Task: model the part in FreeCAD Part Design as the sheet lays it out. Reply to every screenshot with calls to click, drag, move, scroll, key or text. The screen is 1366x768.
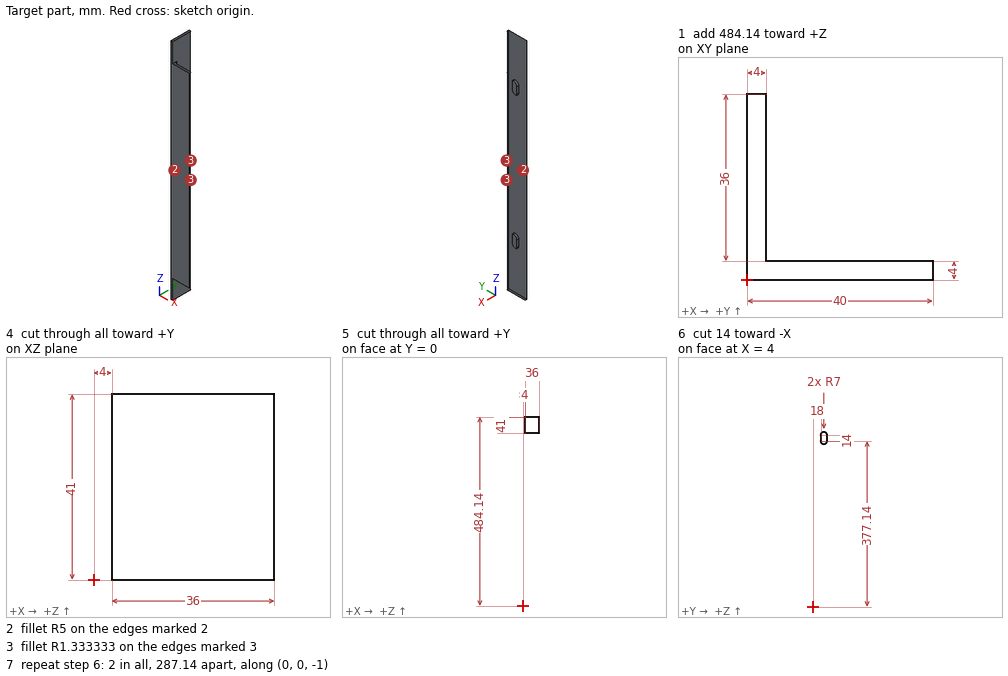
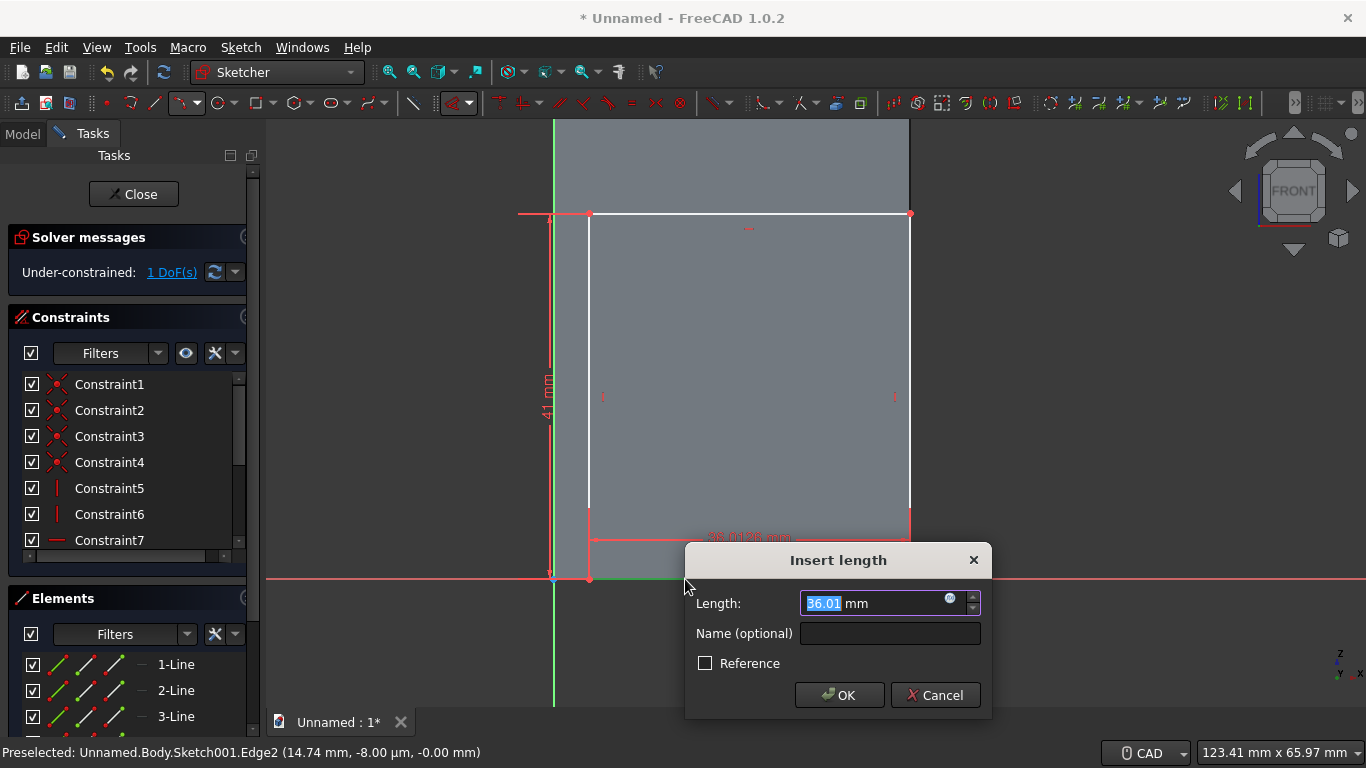
text(36)
key(Return)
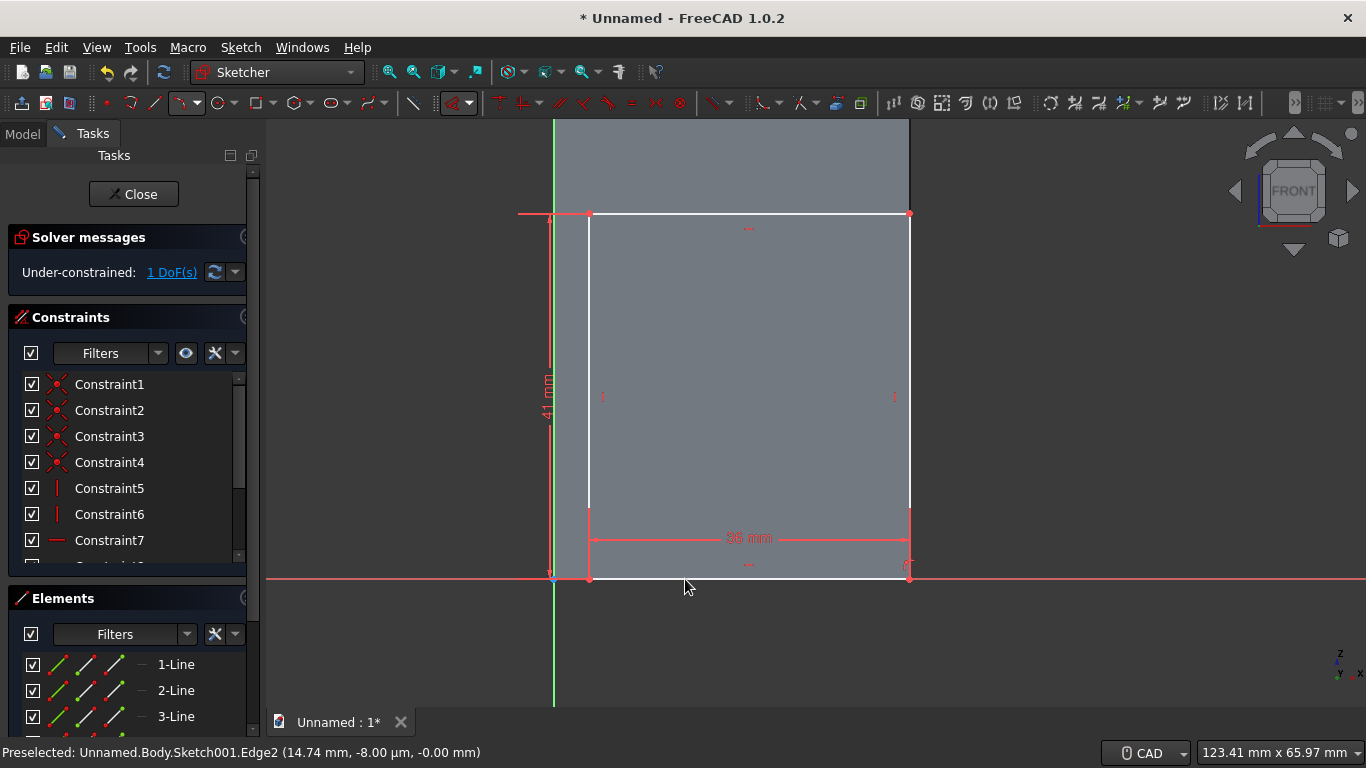
click(589, 214)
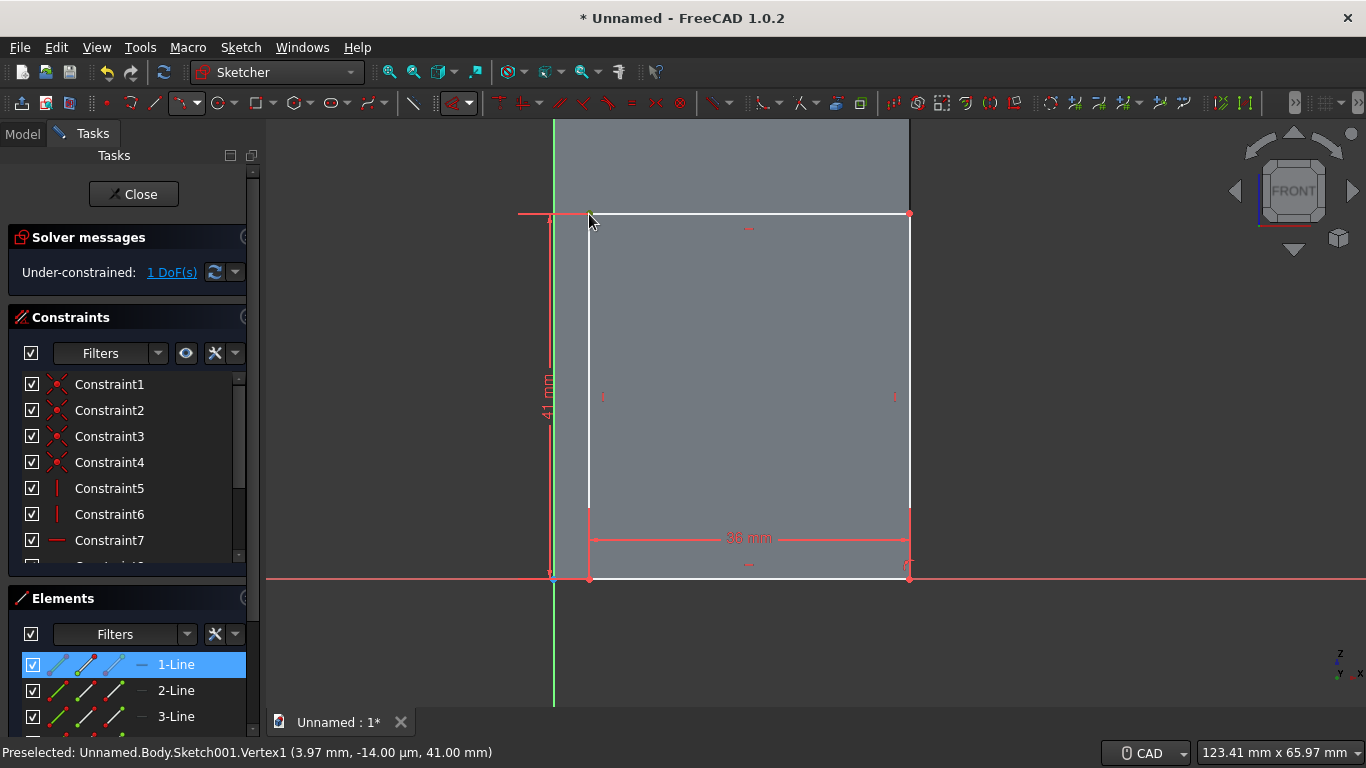
click(472, 104)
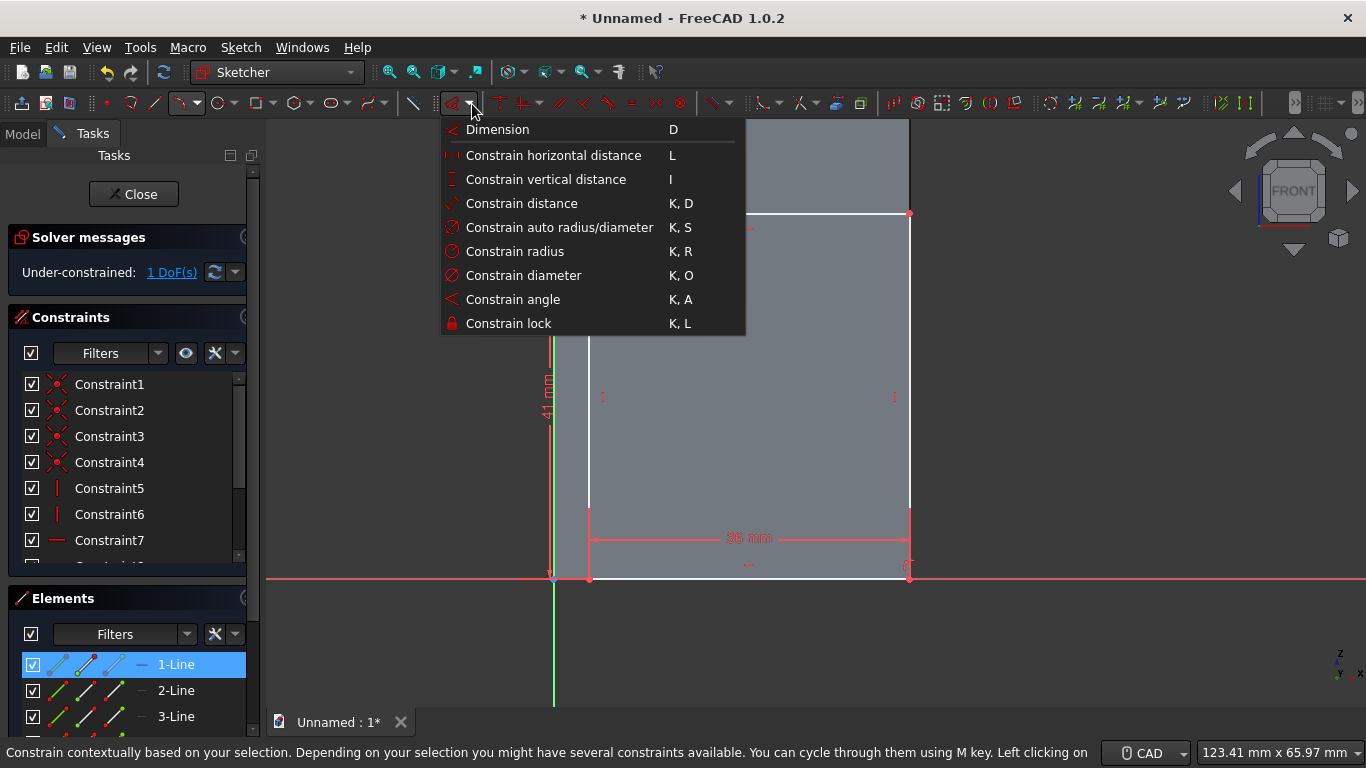
click(593, 155)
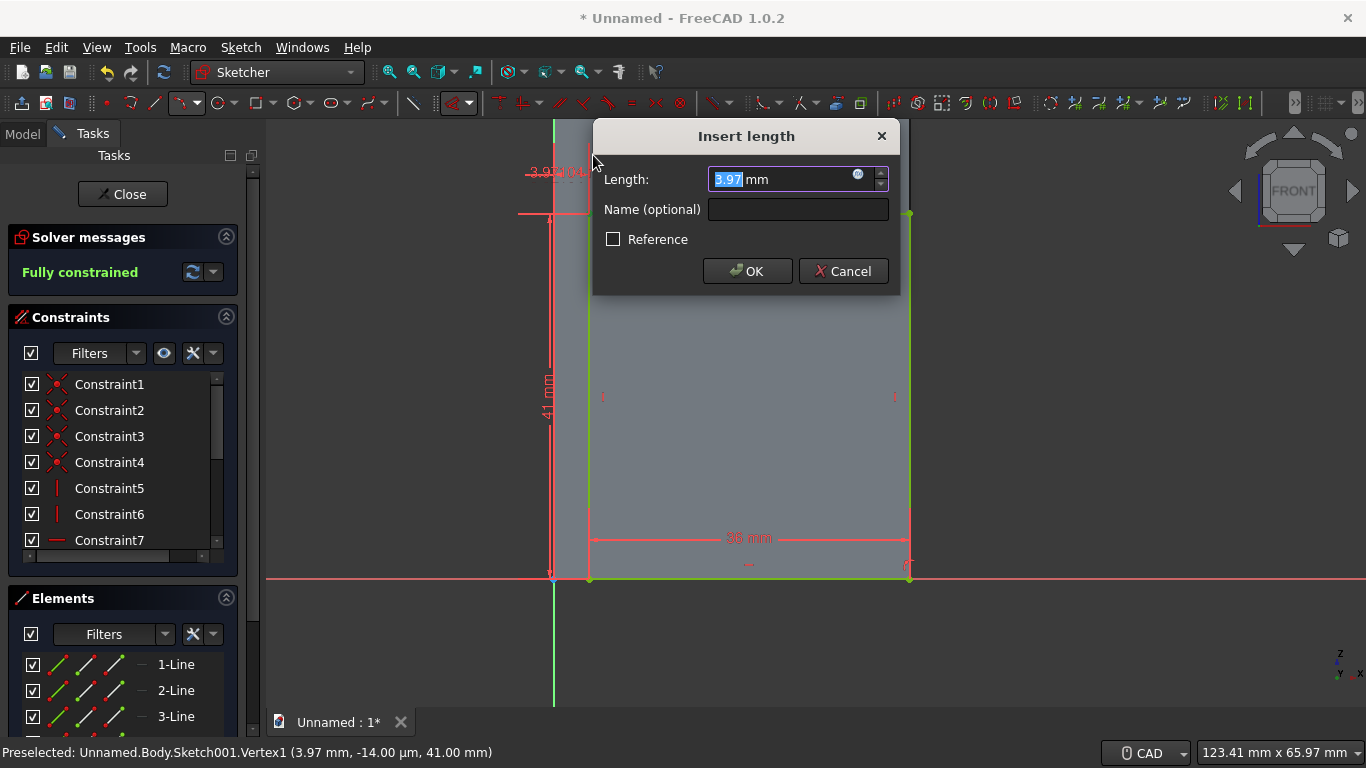
text(4)
key(Return)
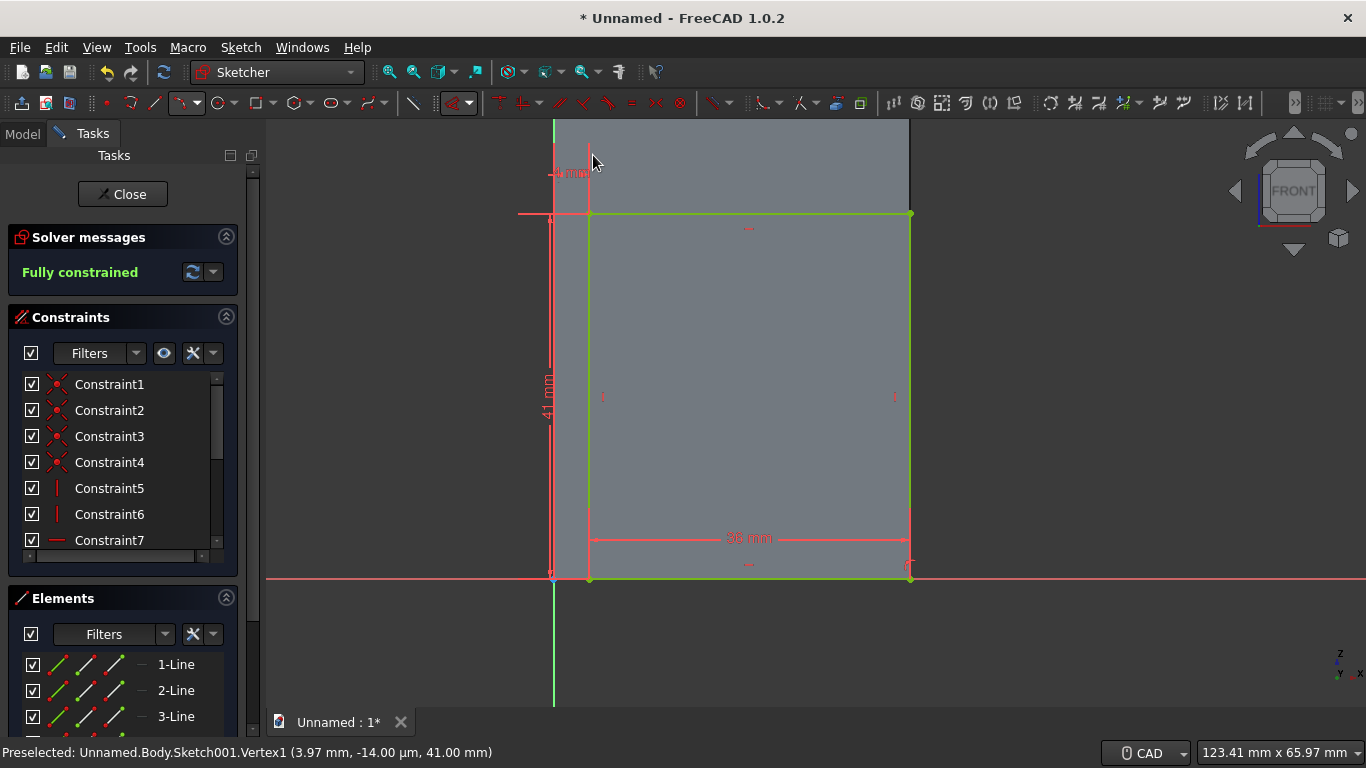
click(123, 194)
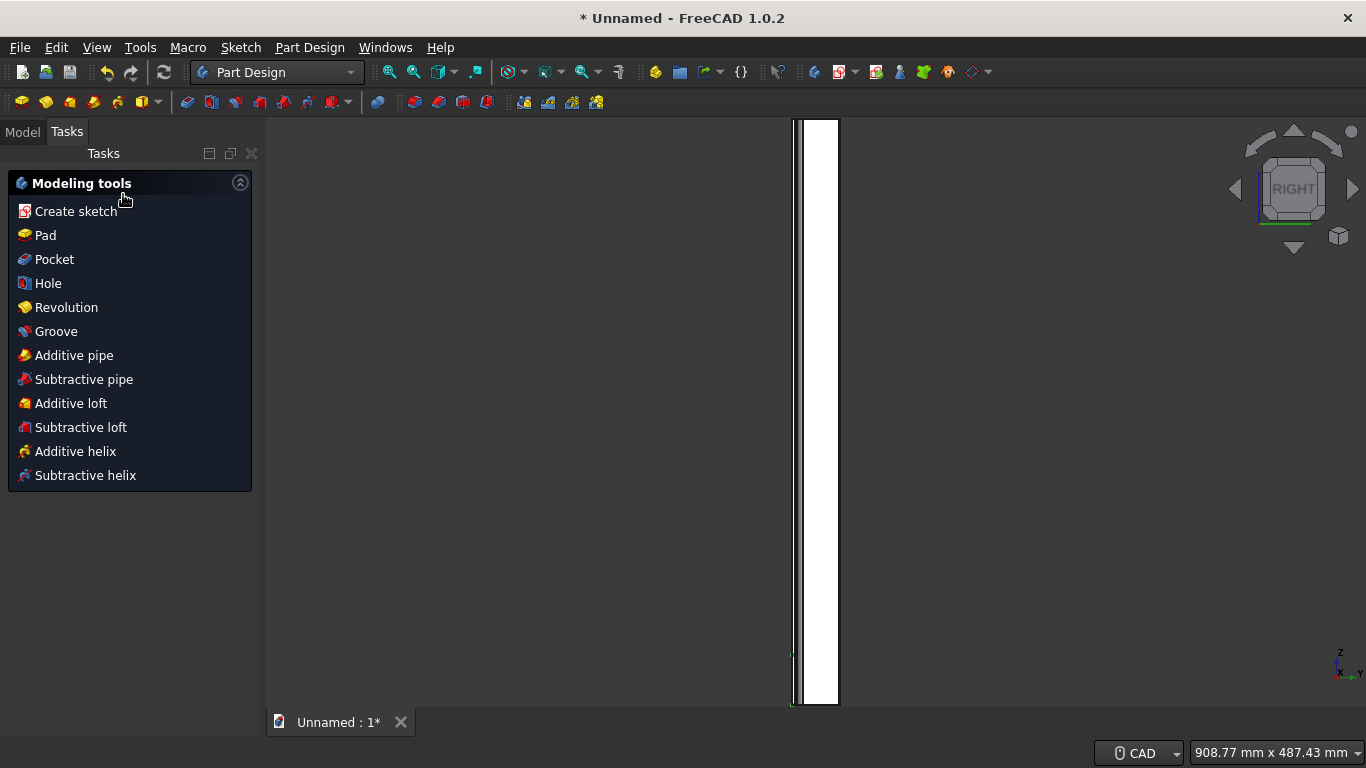
click(188, 102)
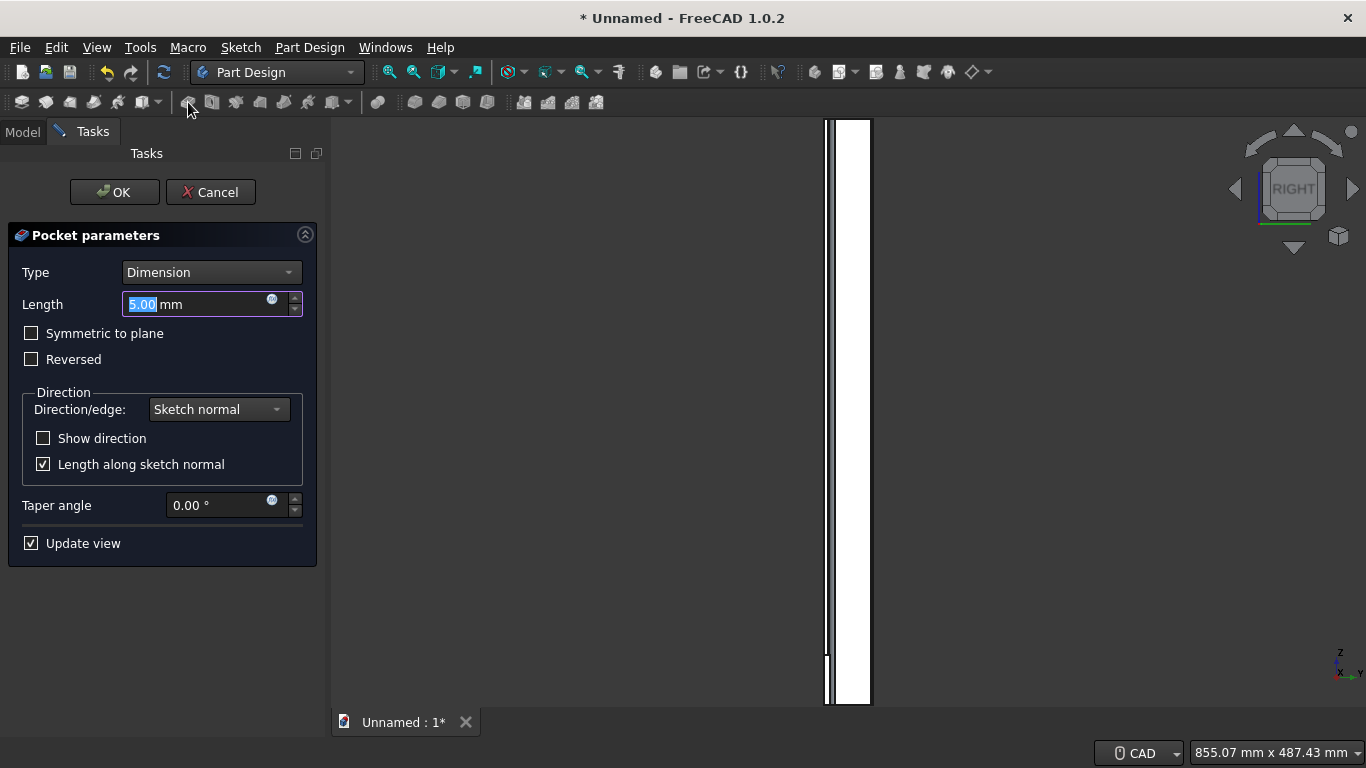
click(212, 272)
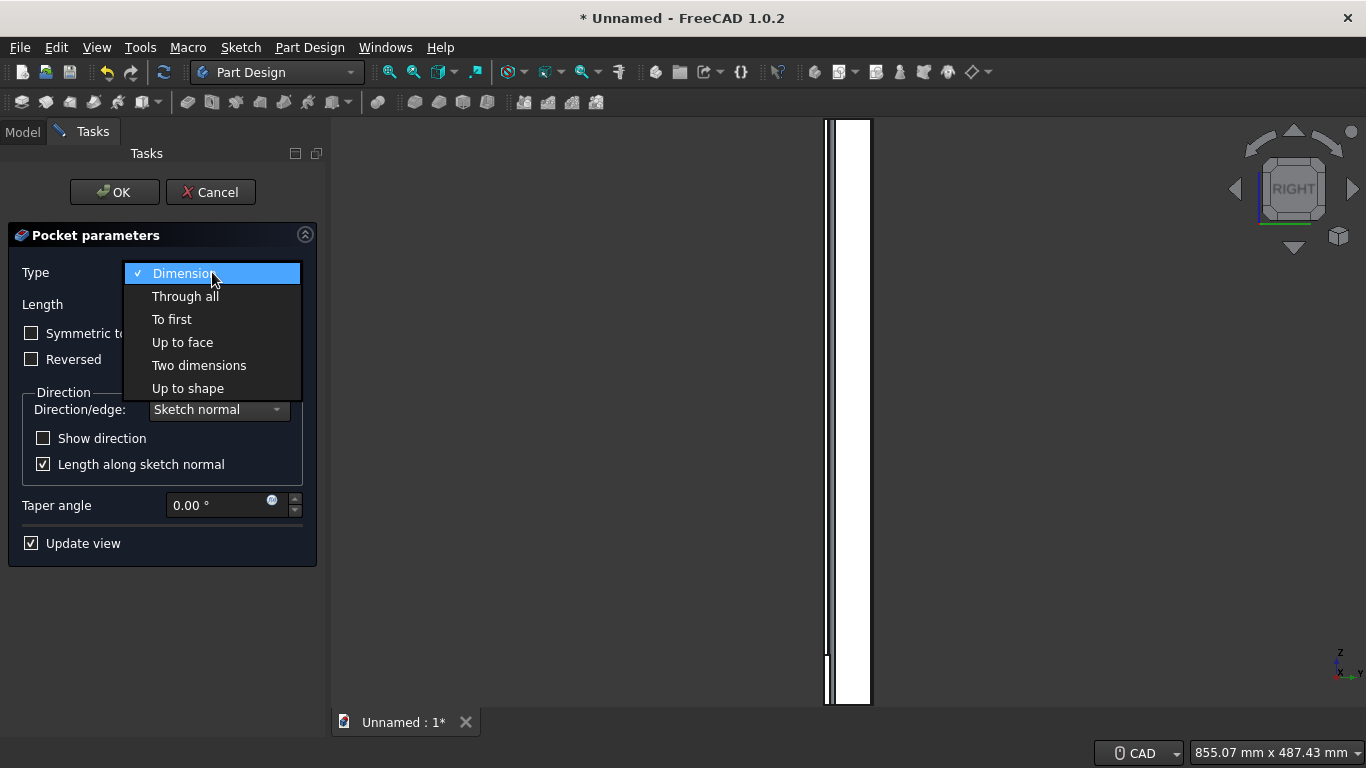
click(212, 296)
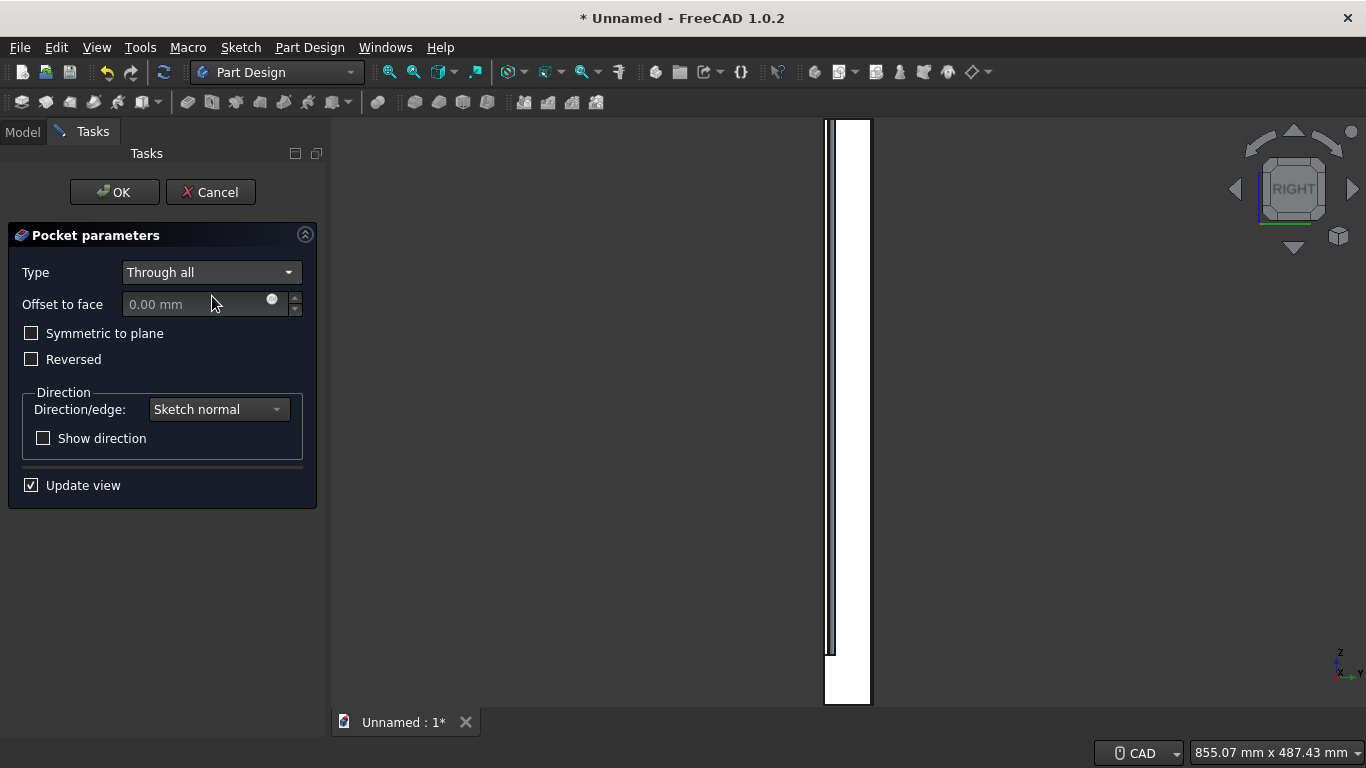
click(115, 192)